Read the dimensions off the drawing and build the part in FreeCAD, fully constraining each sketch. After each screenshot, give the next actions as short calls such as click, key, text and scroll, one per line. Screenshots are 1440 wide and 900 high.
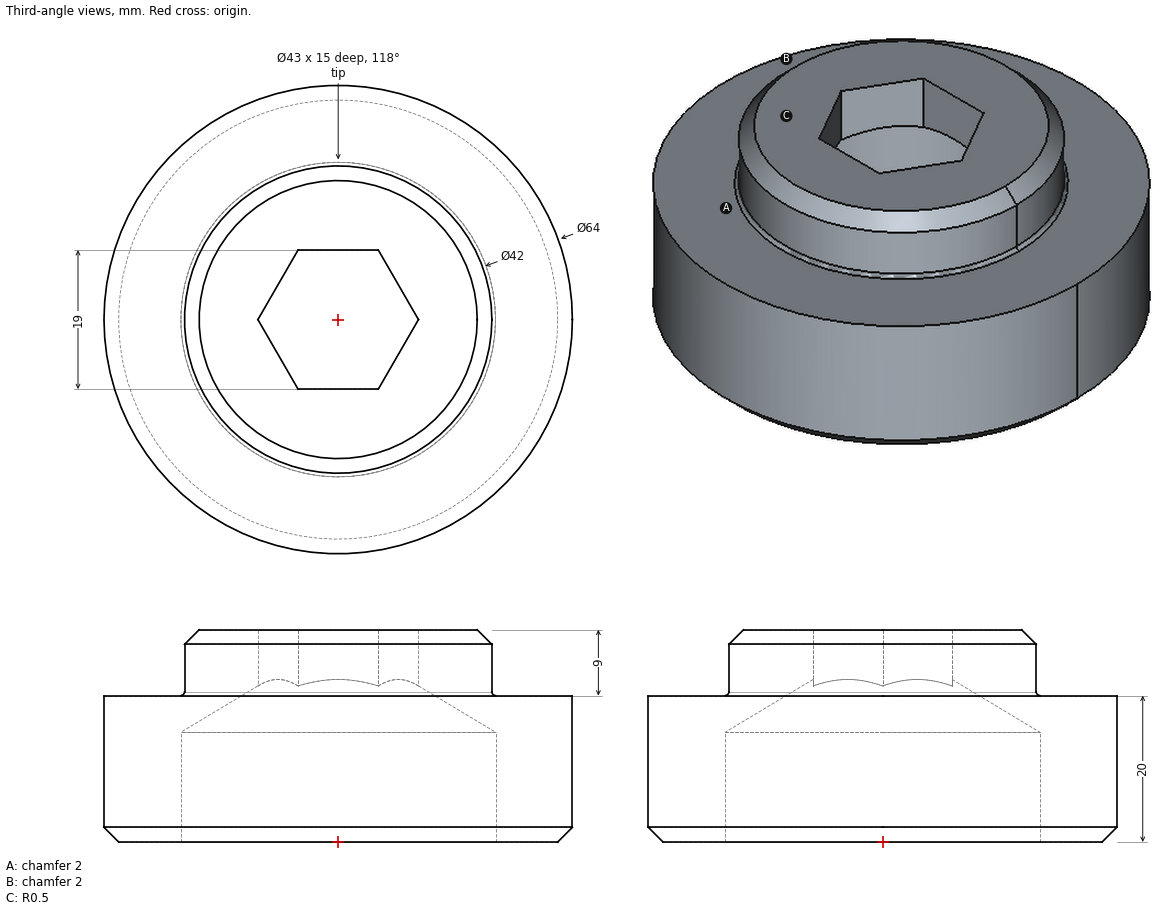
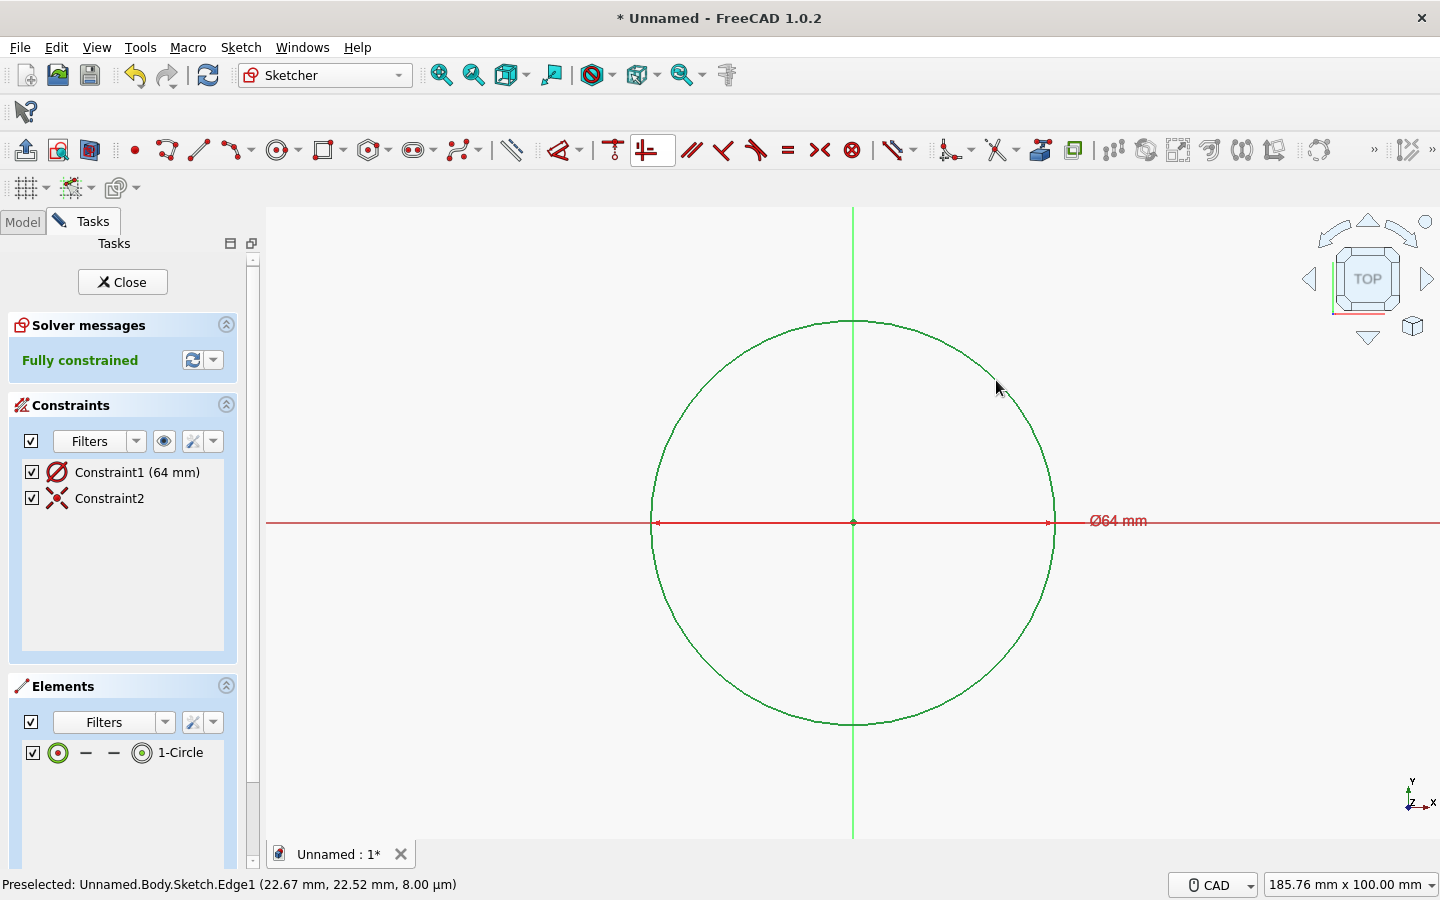
click(123, 282)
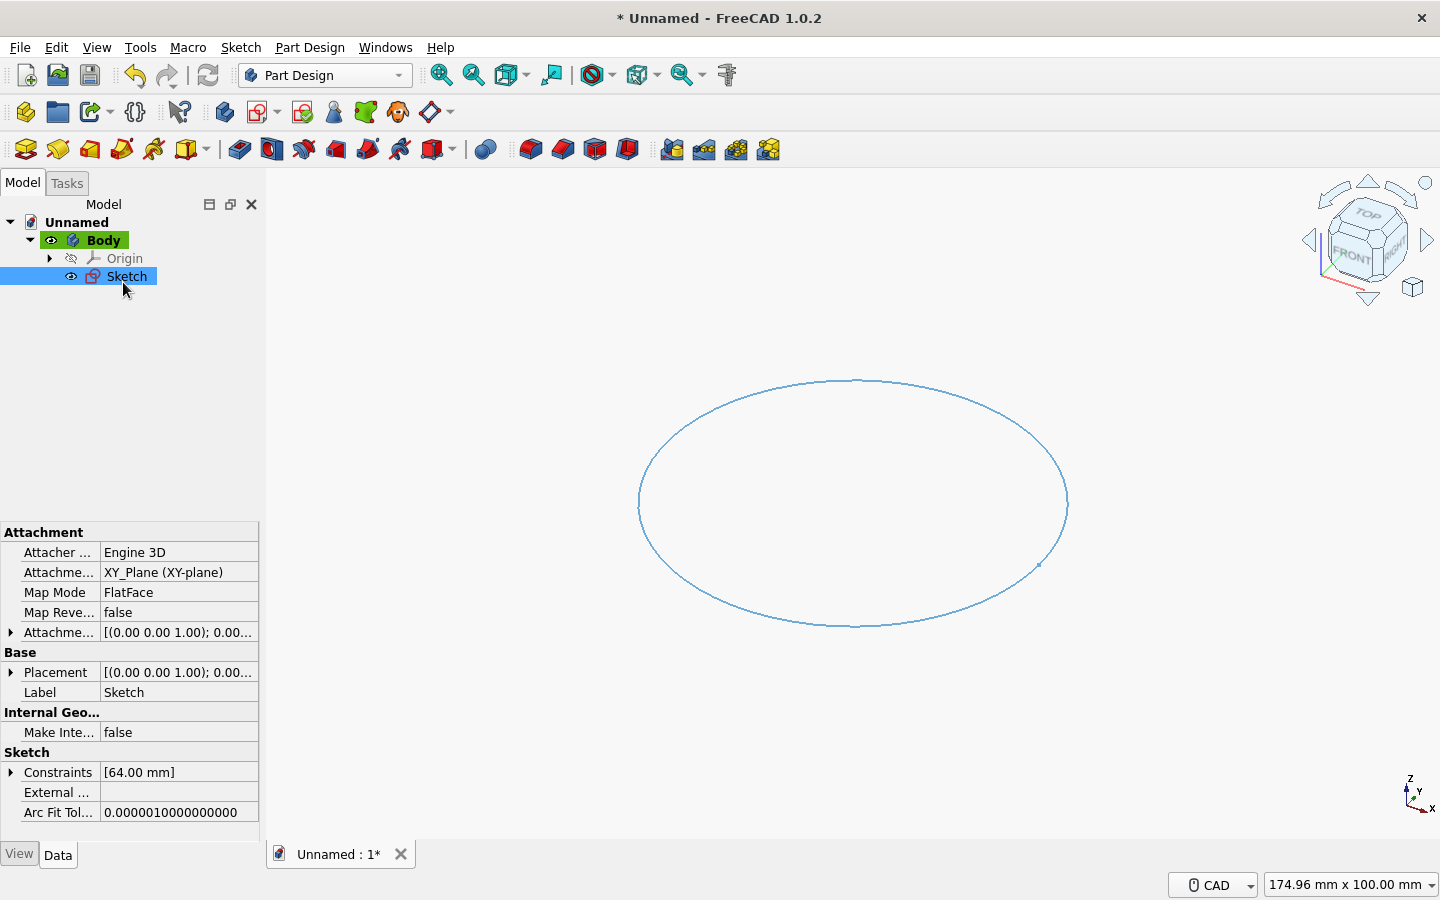
click(26, 150)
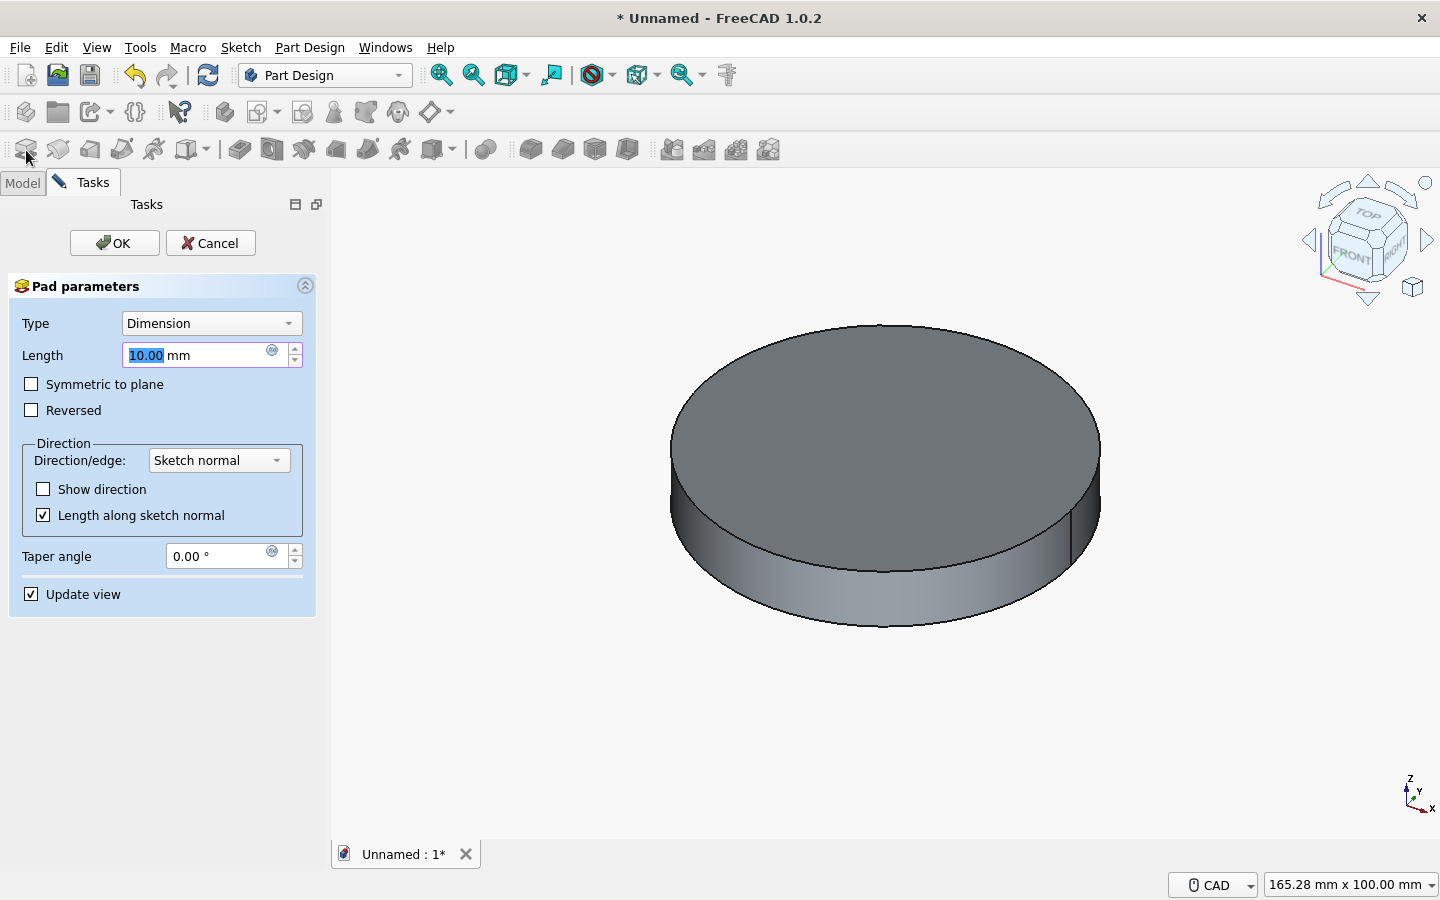
text(20)
key(Tab)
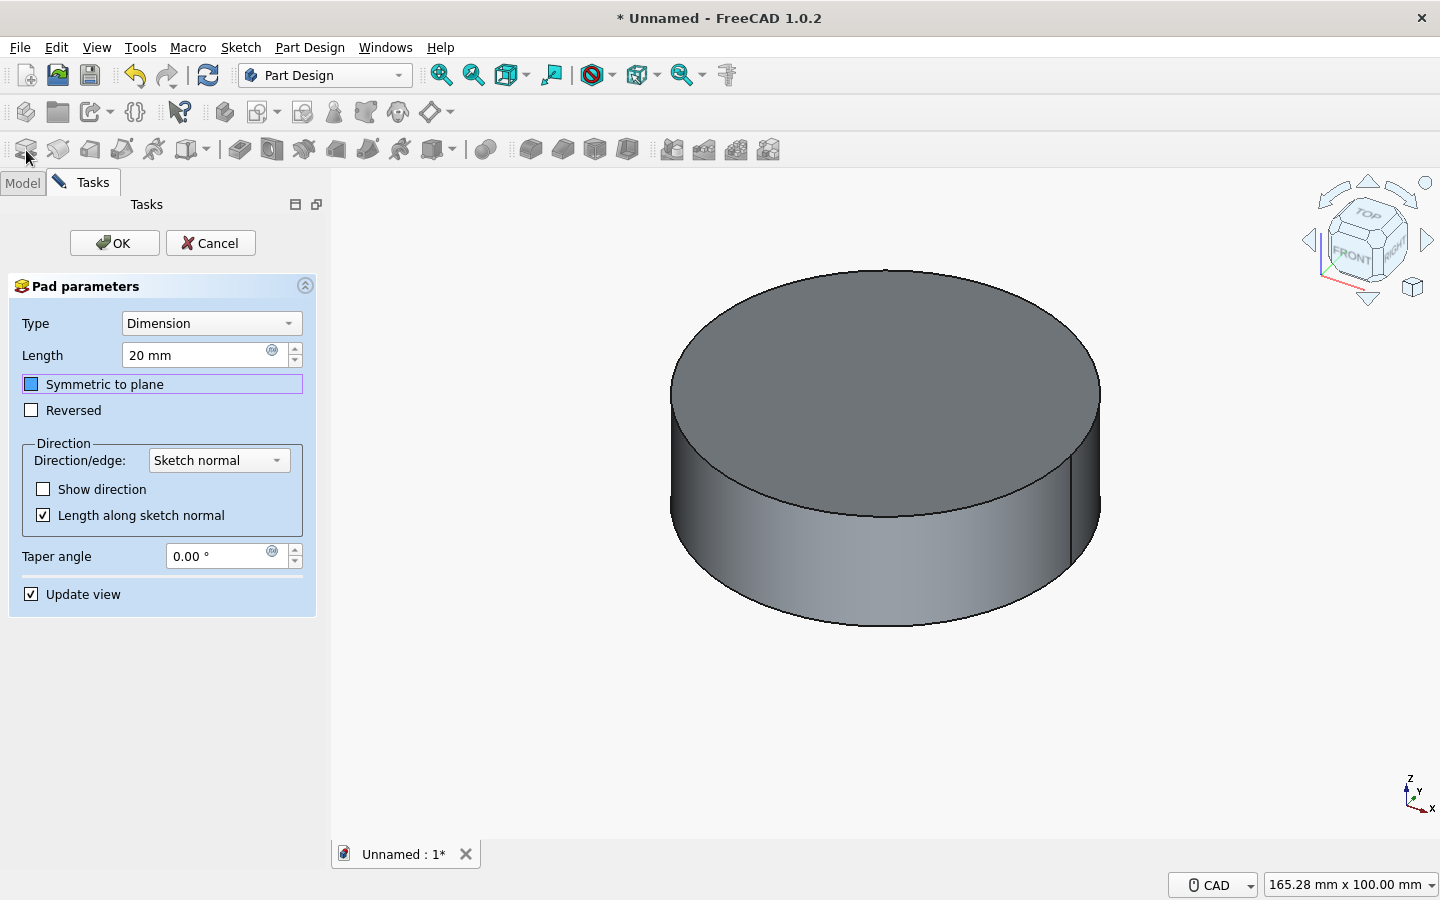
click(115, 243)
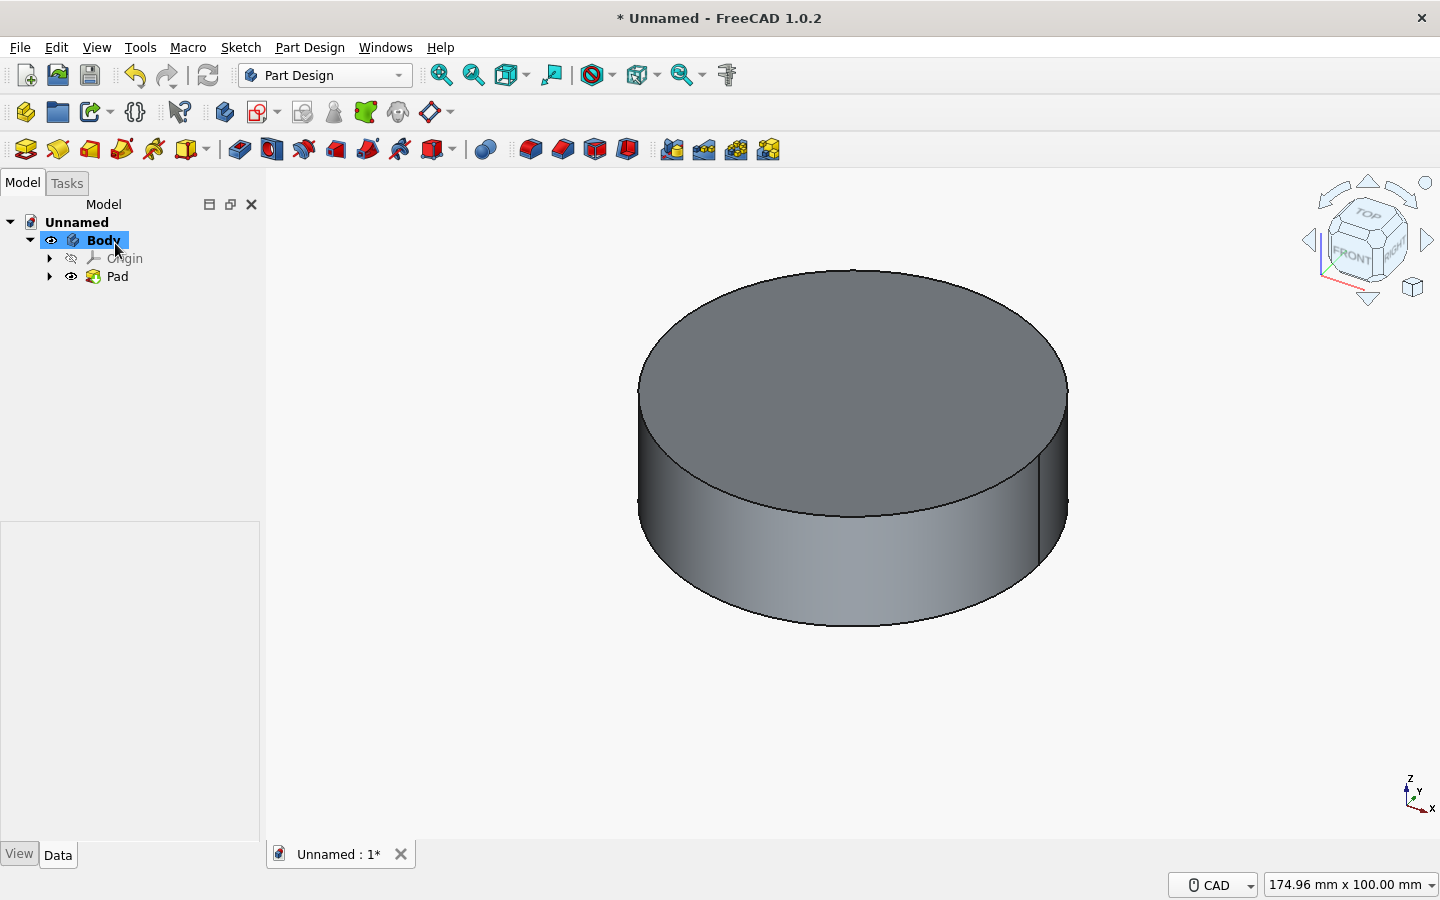
click(853, 393)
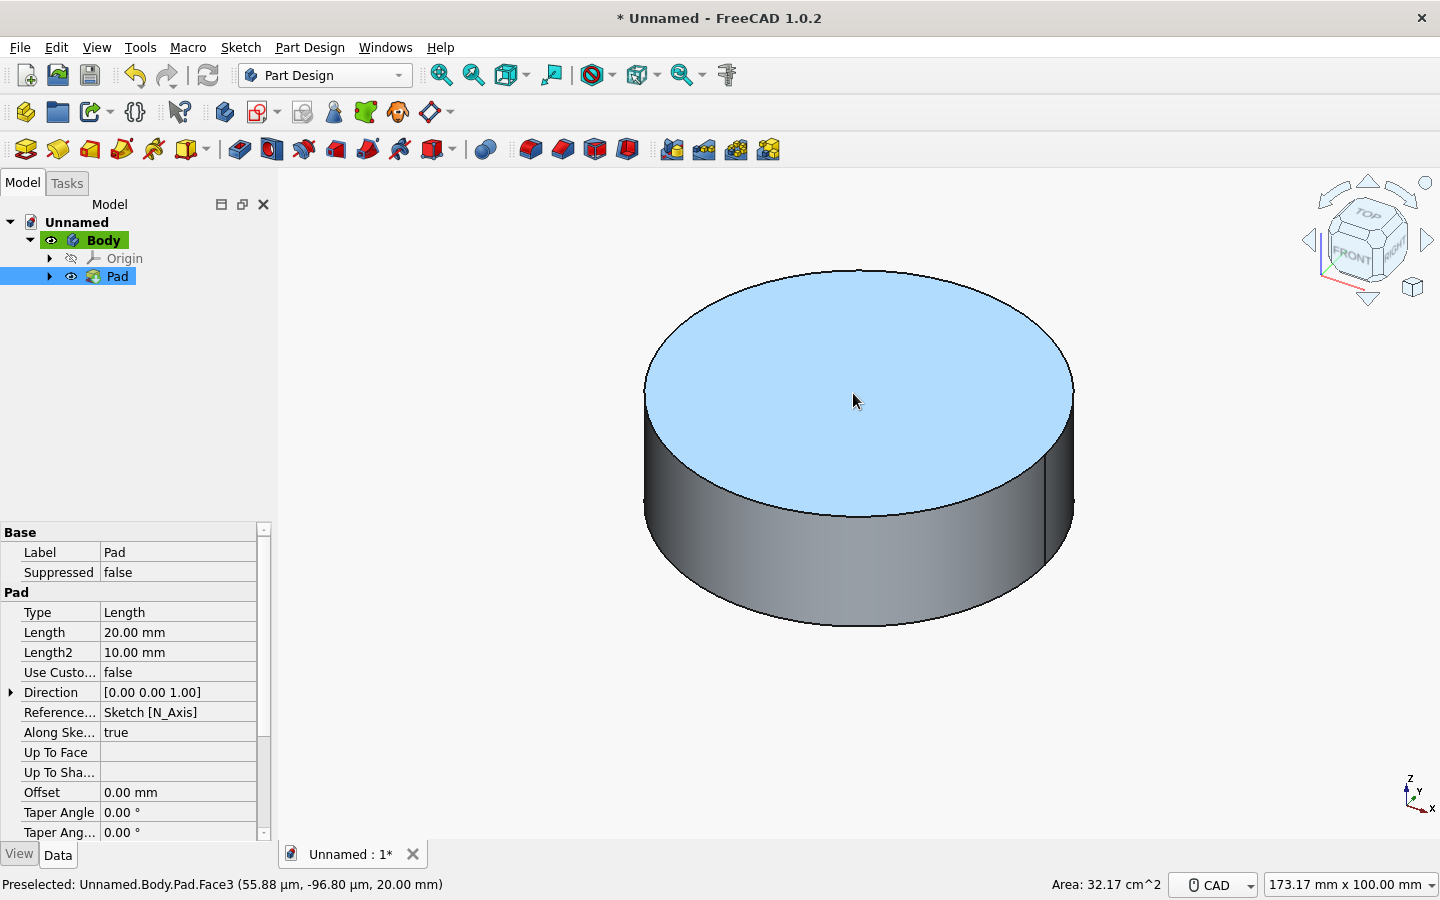
click(258, 112)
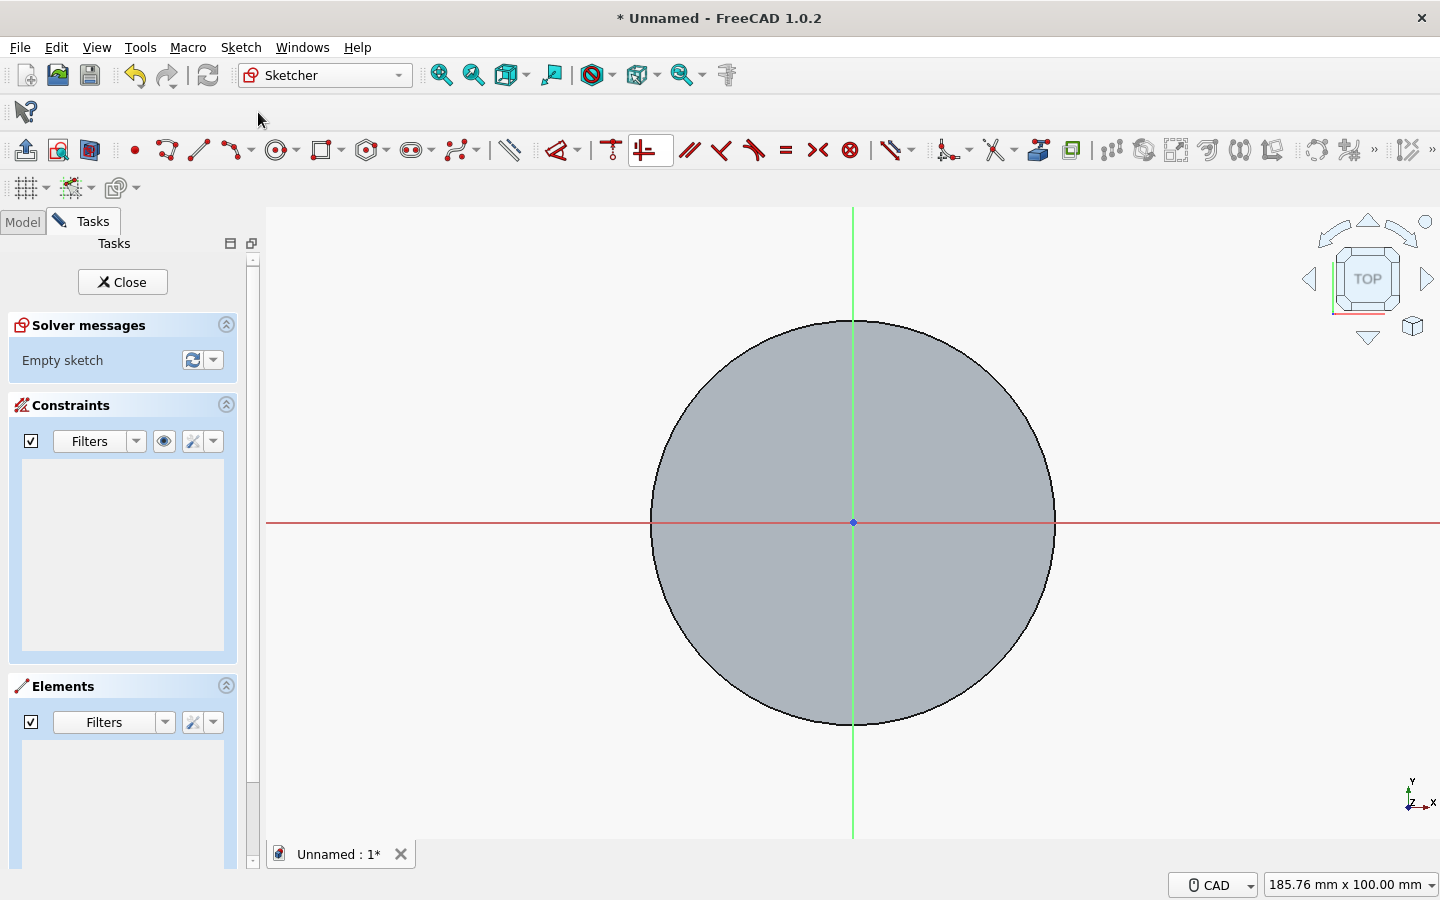
scroll(992, 523, up, 2)